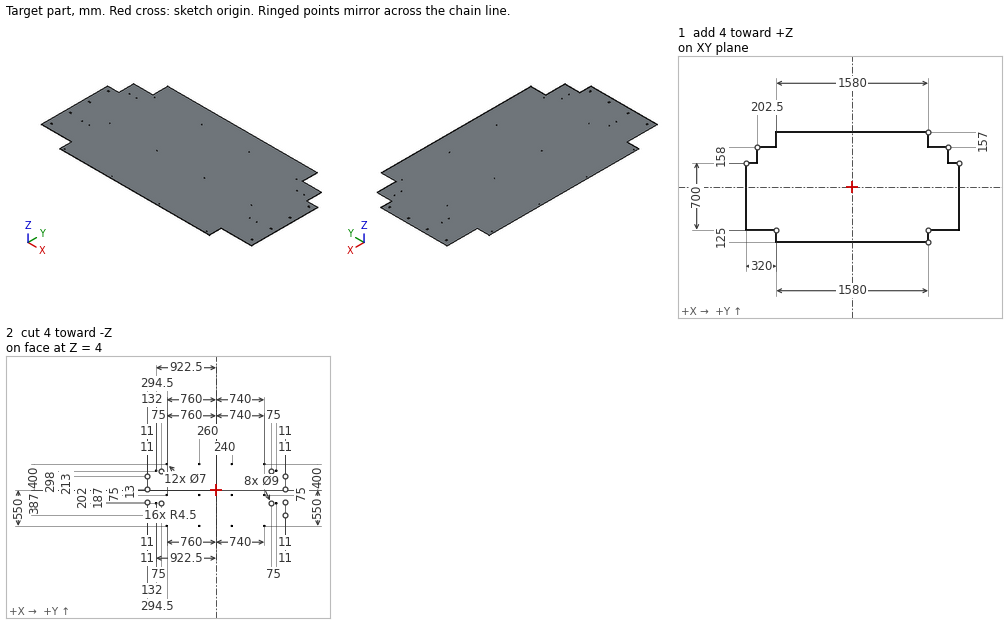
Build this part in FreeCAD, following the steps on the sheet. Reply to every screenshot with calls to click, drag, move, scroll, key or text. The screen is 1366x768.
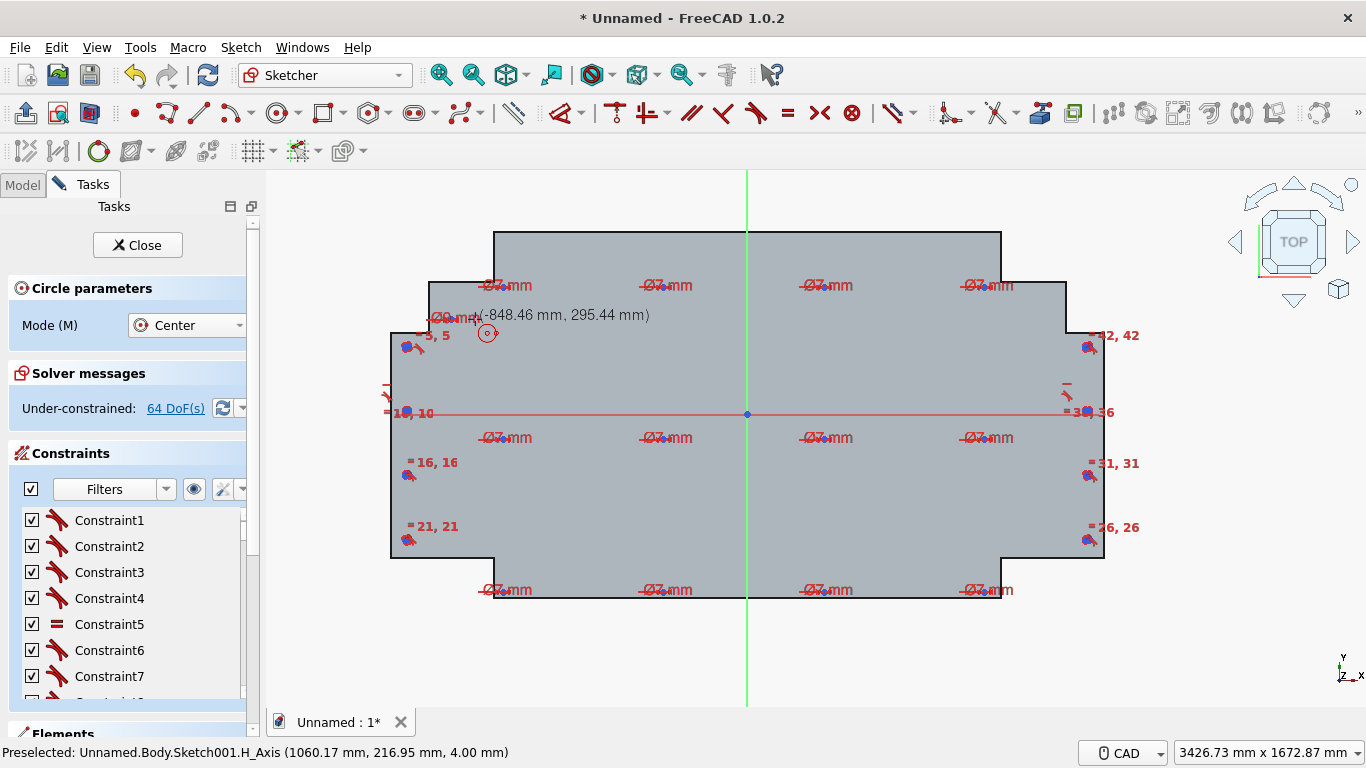
click(475, 319)
move(476, 318)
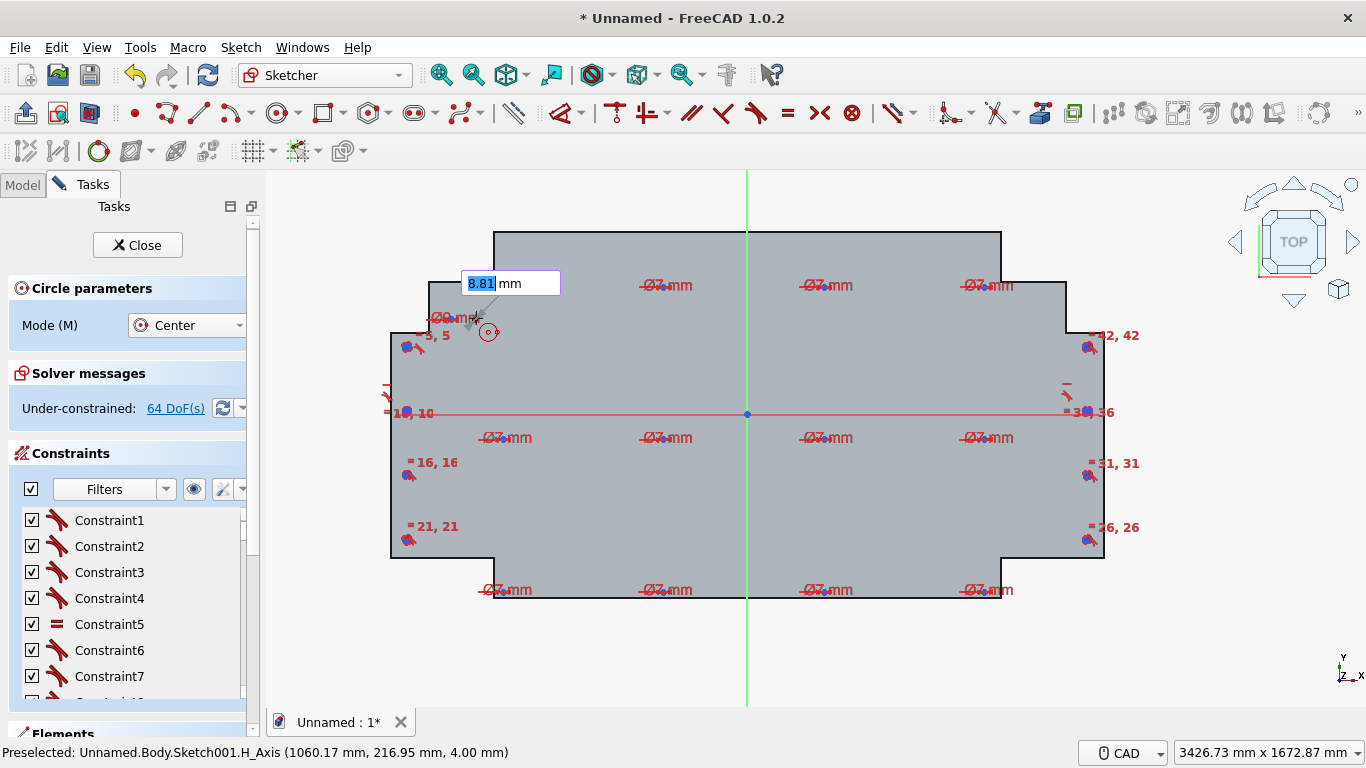
text(9)
key(Return)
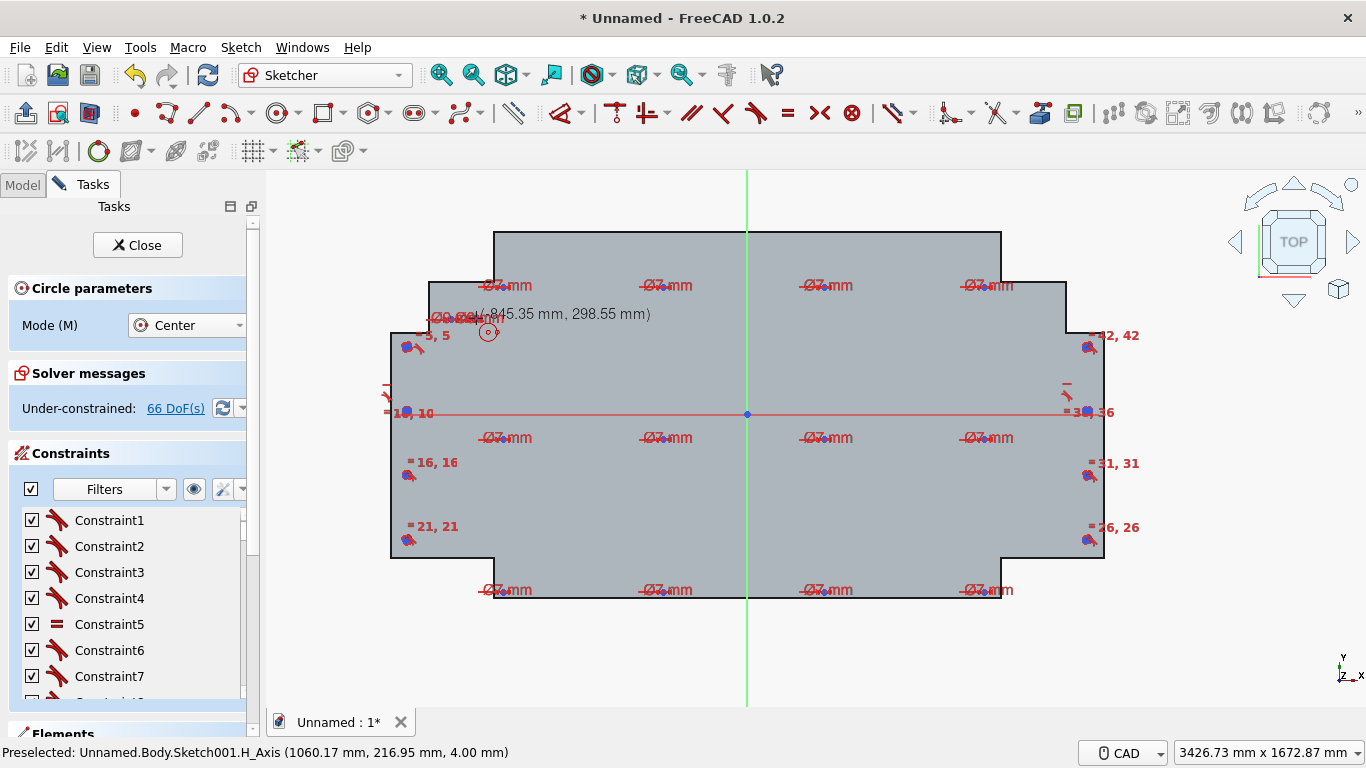
scroll(451, 480, up, 14)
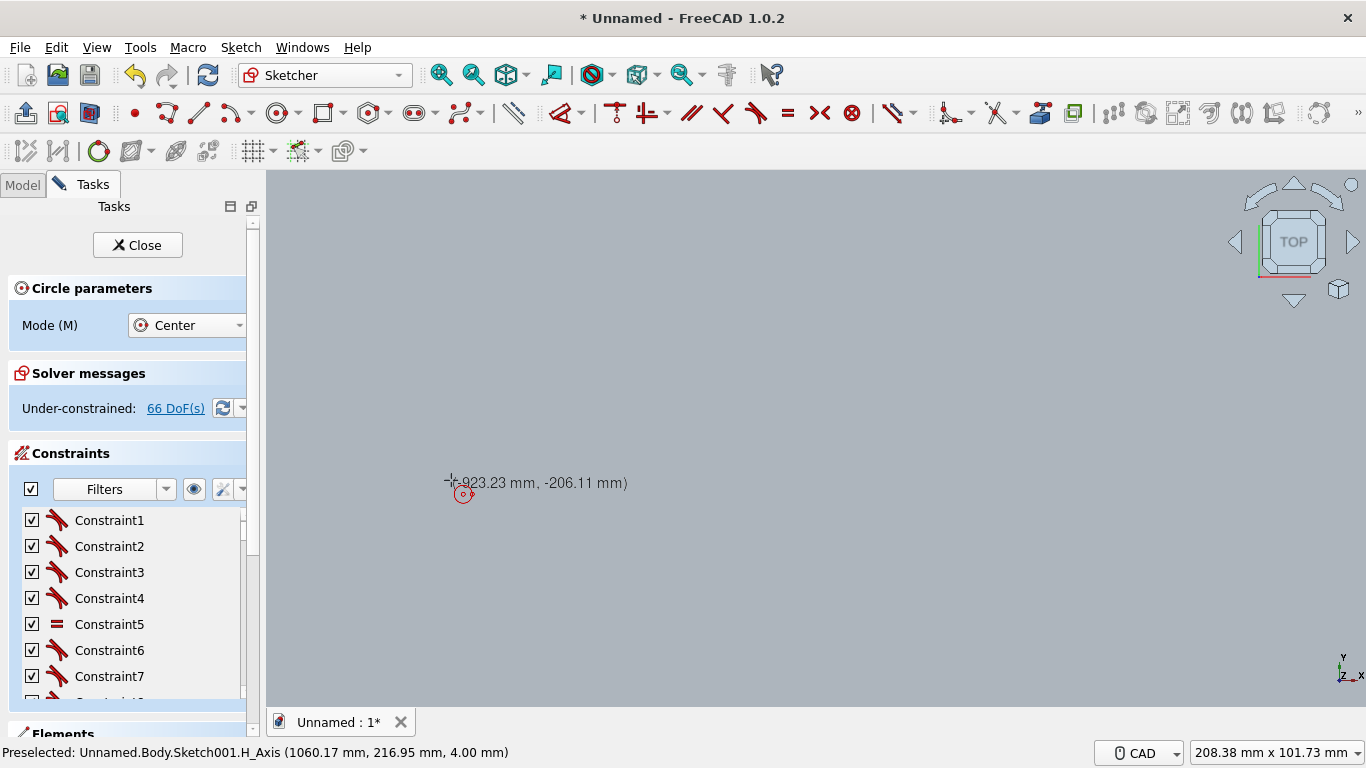
scroll(451, 480, down, 14)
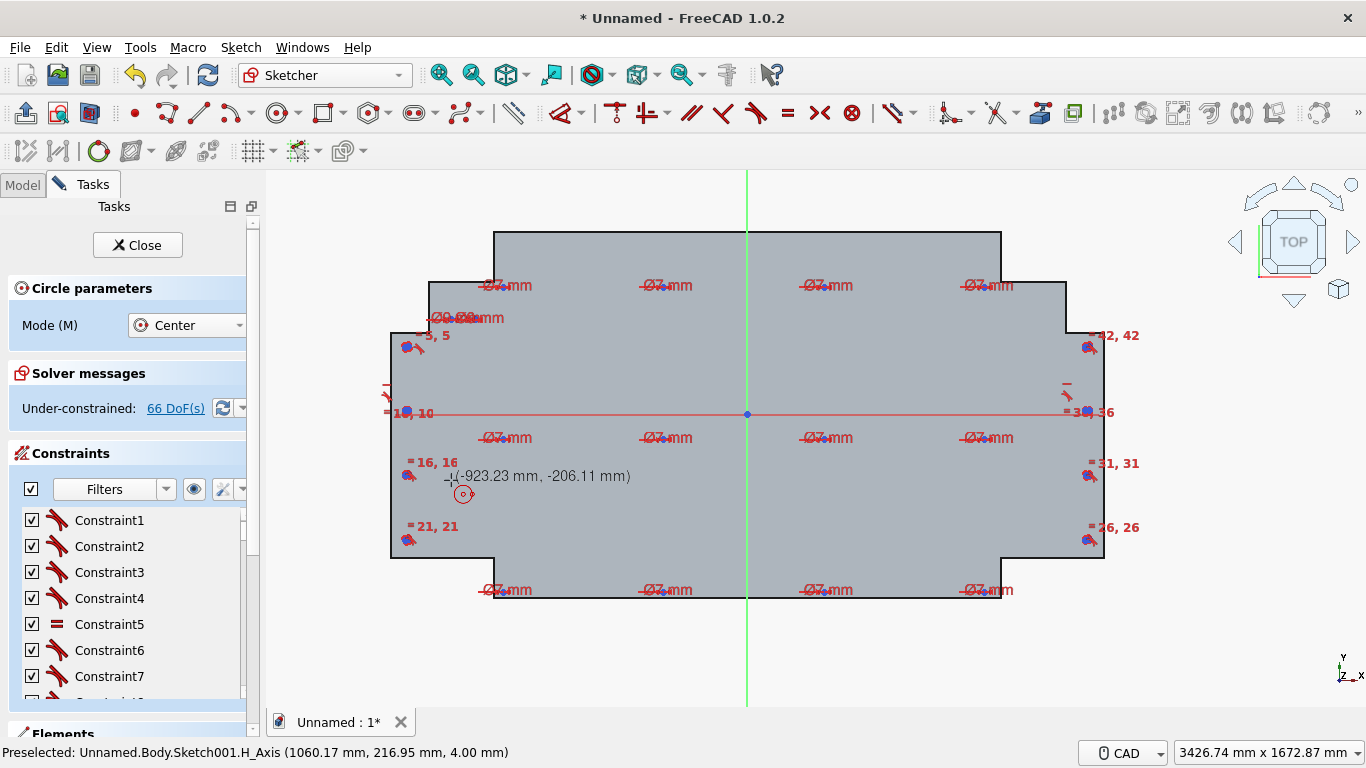
click(451, 480)
move(452, 479)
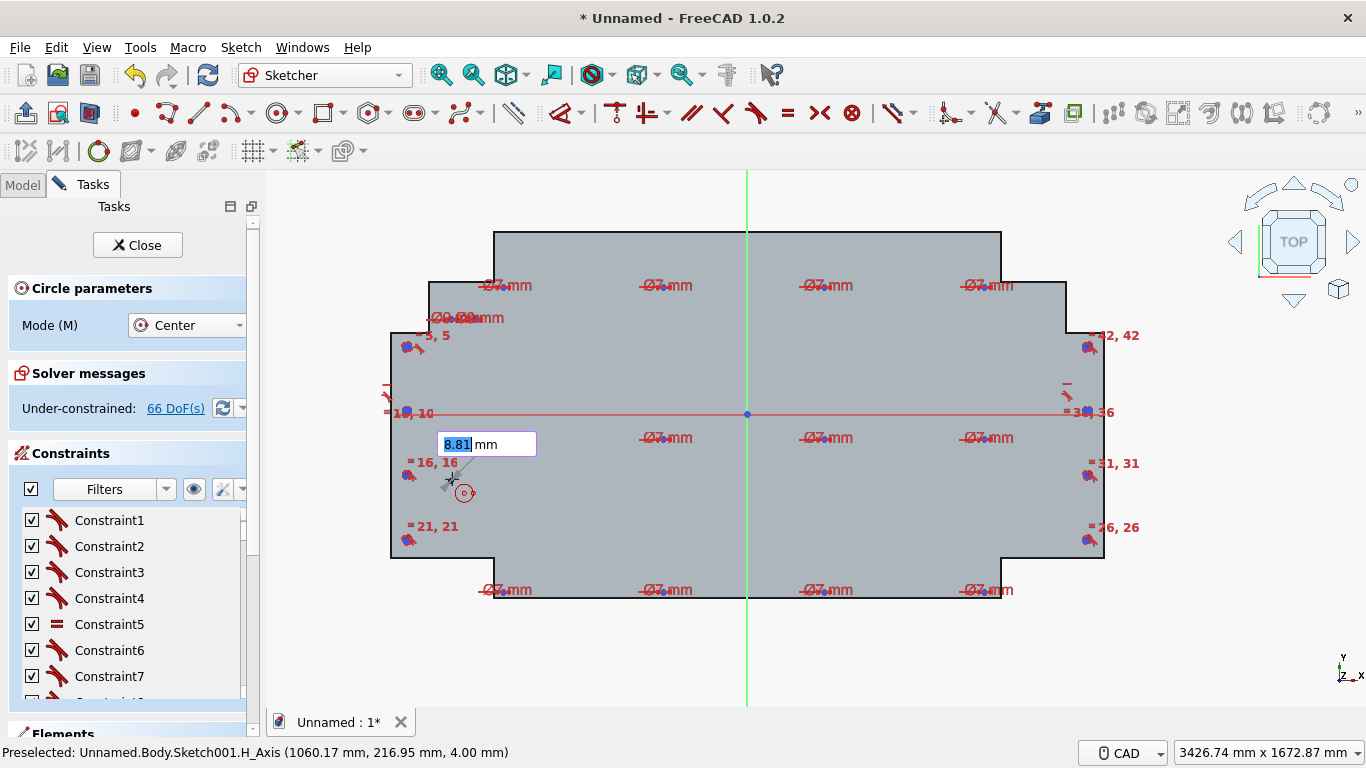
text(9)
key(Return)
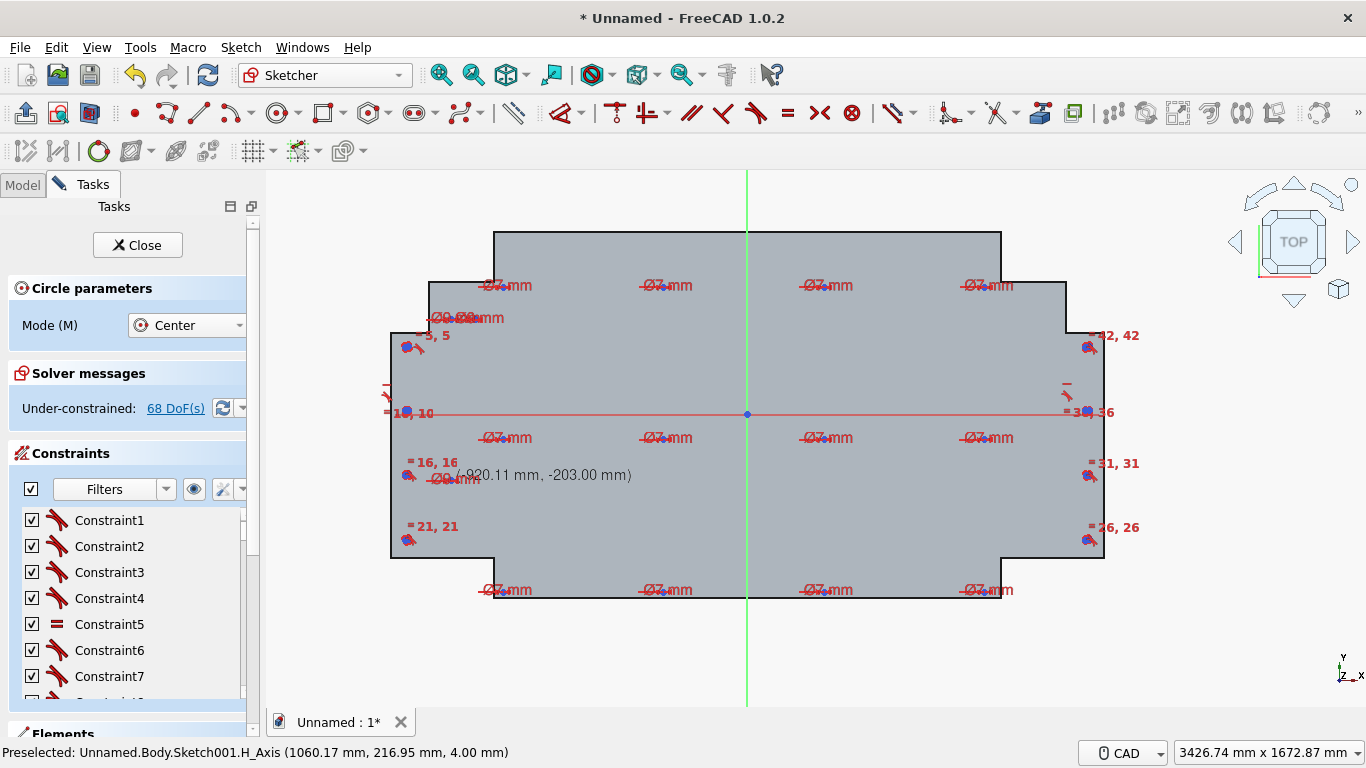
scroll(475, 480, up, 14)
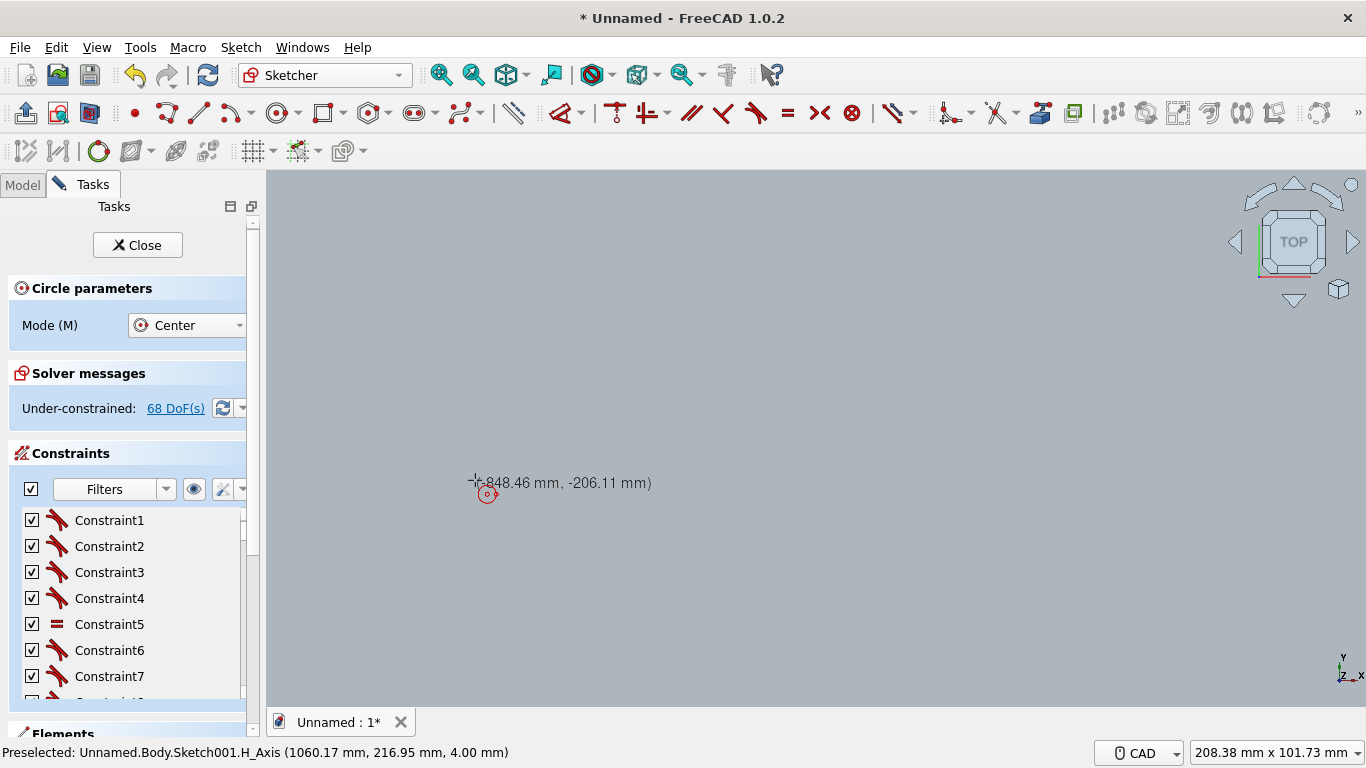
scroll(475, 480, down, 14)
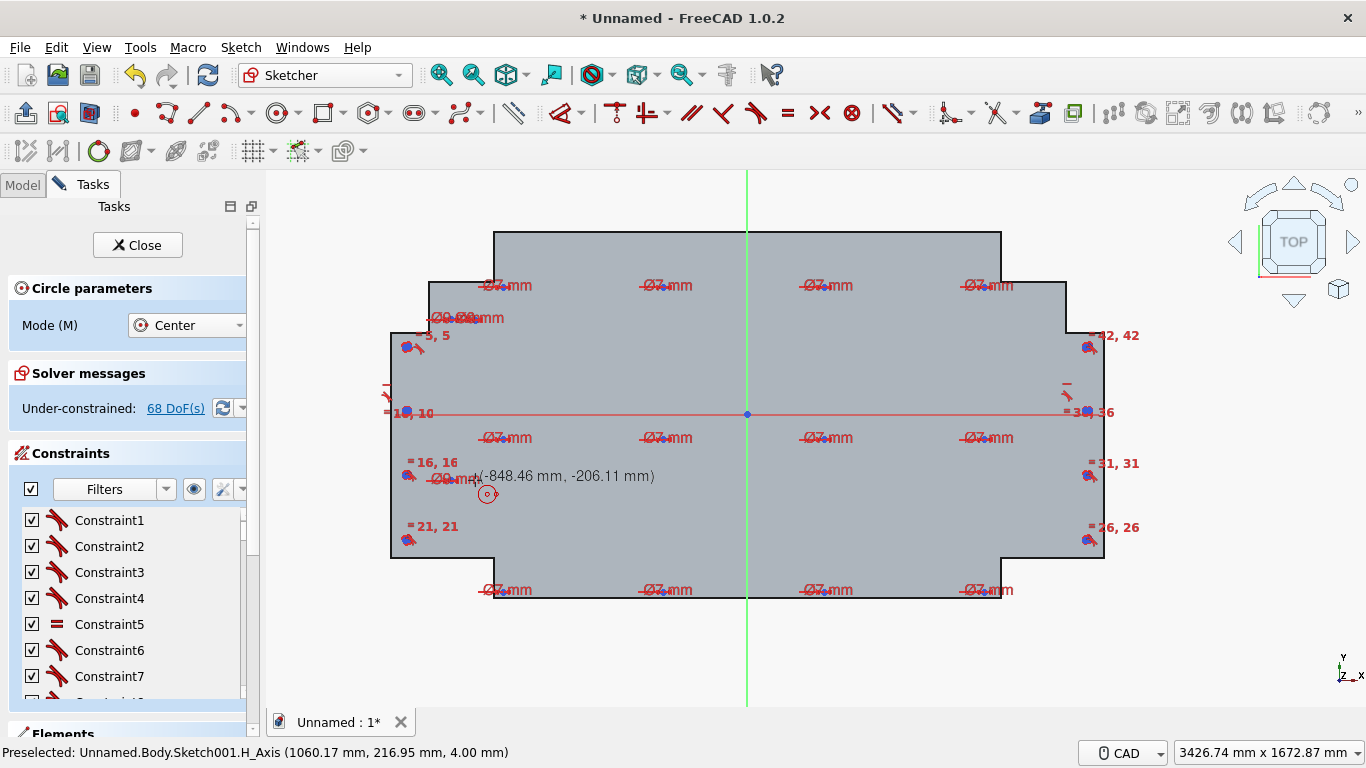
click(475, 480)
move(476, 479)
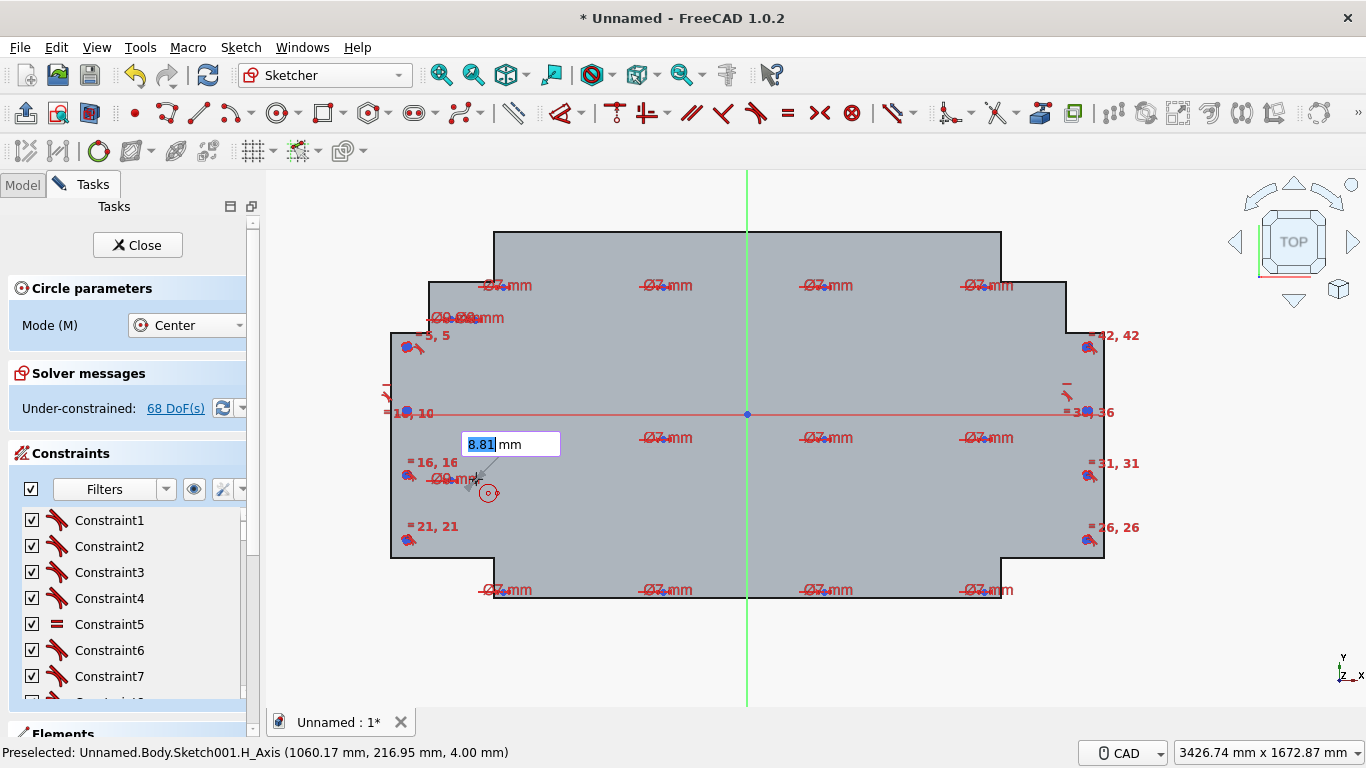
text(9)
key(Return)